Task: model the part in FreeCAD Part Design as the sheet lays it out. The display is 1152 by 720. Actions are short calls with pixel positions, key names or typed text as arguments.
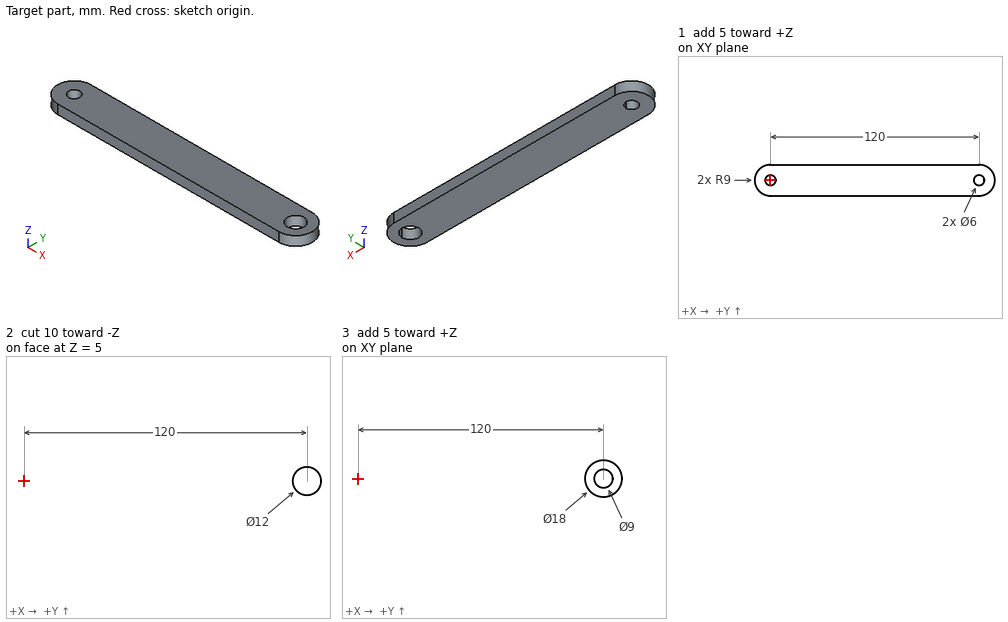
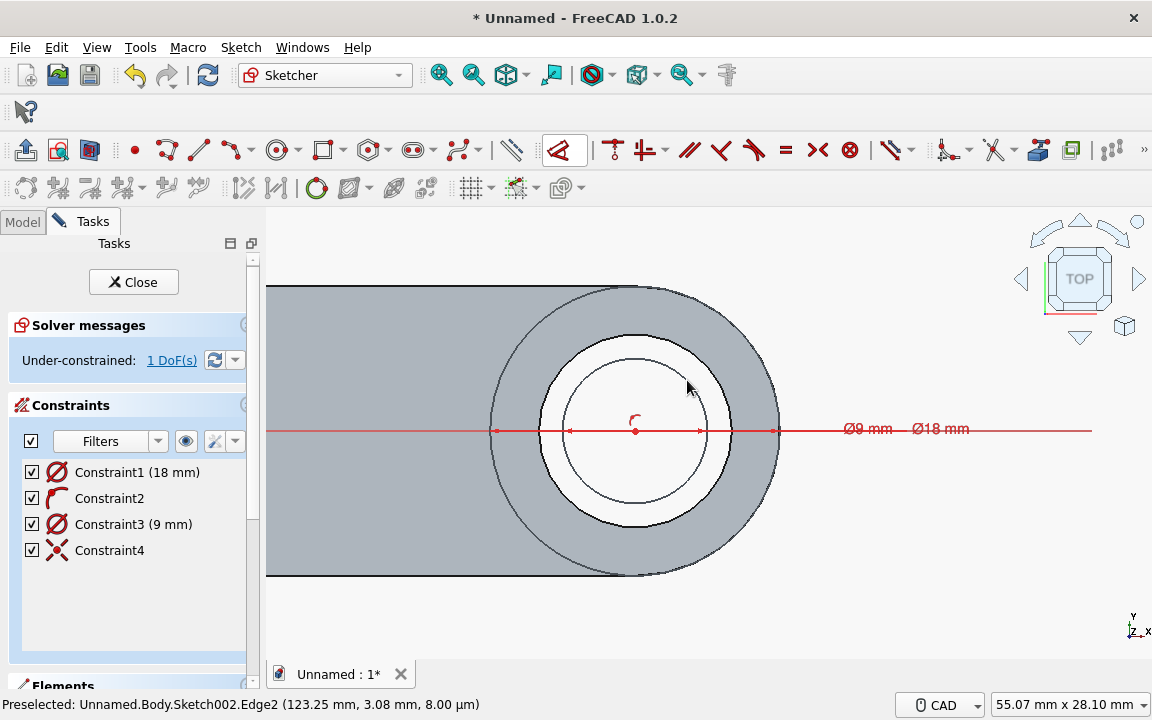
click(635, 431)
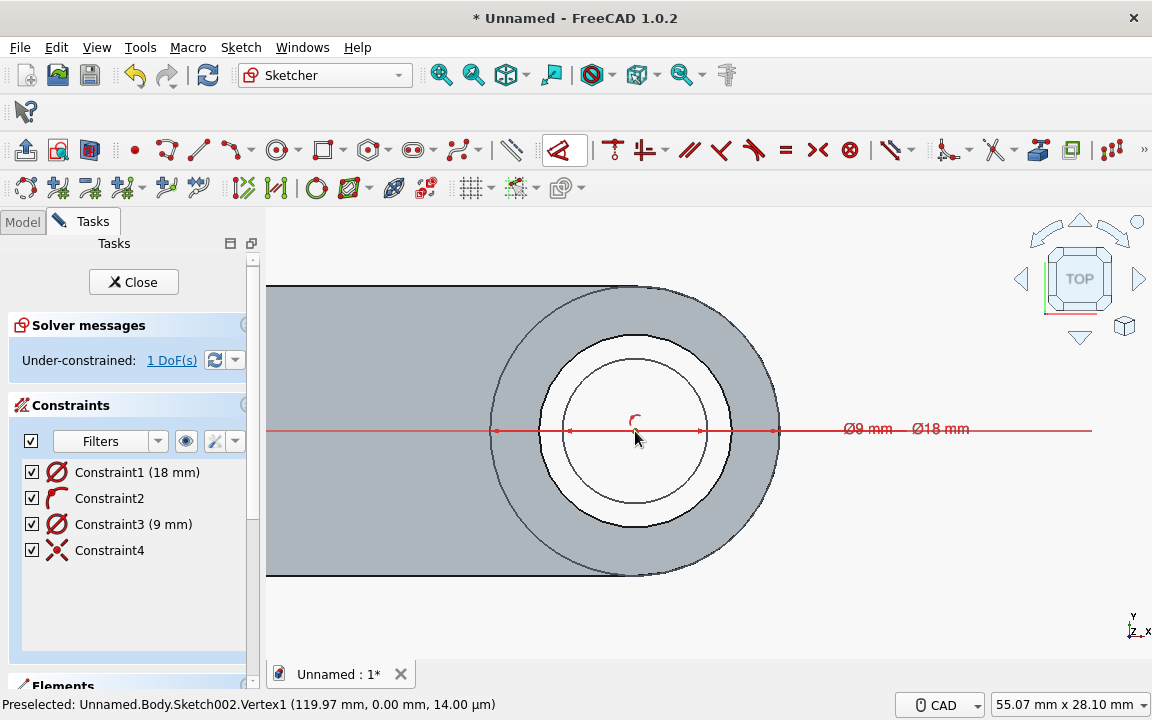
click(582, 150)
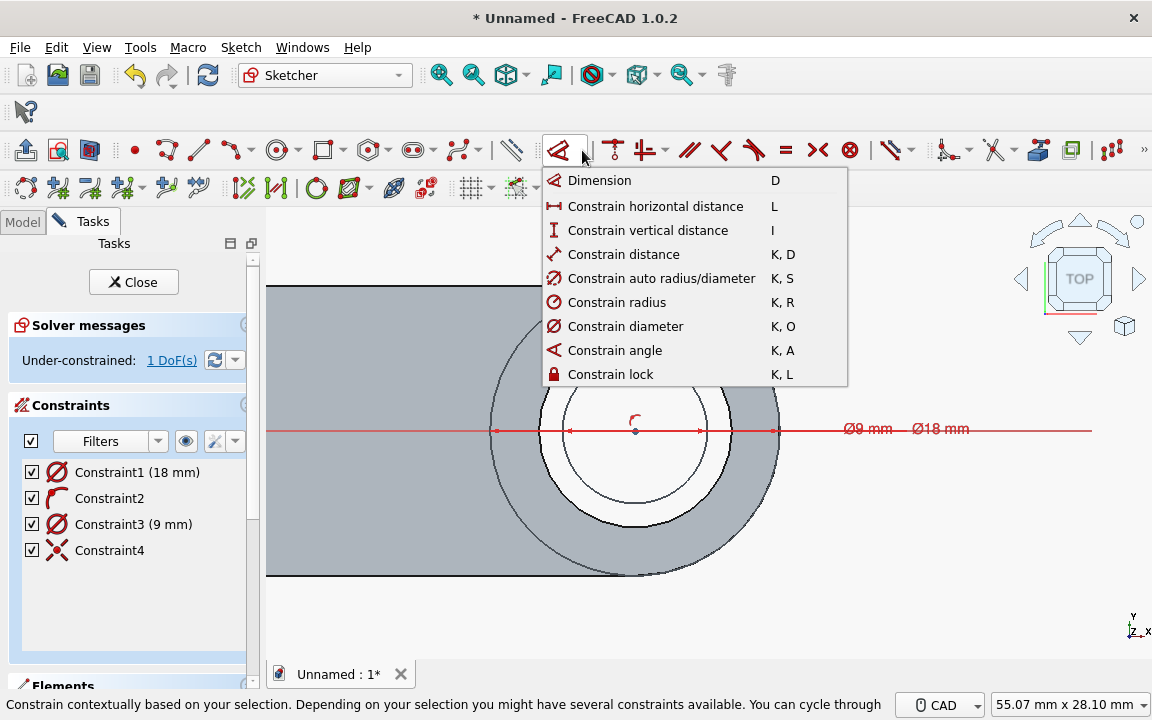
click(695, 206)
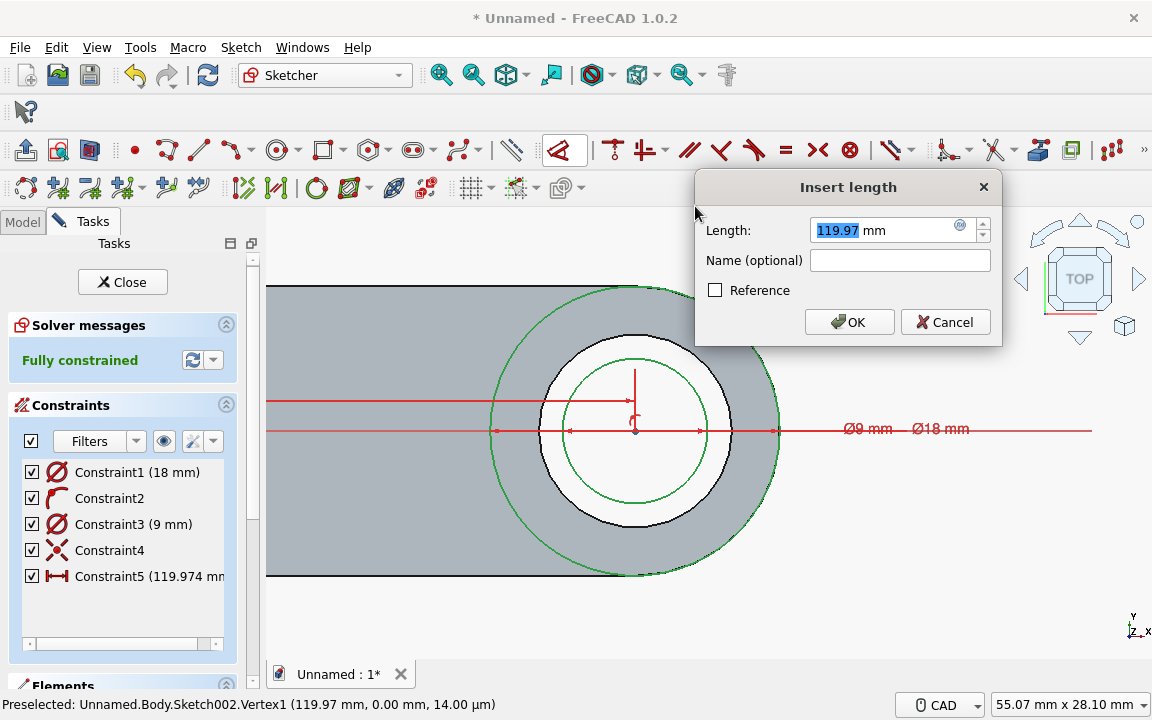
text(120)
key(Return)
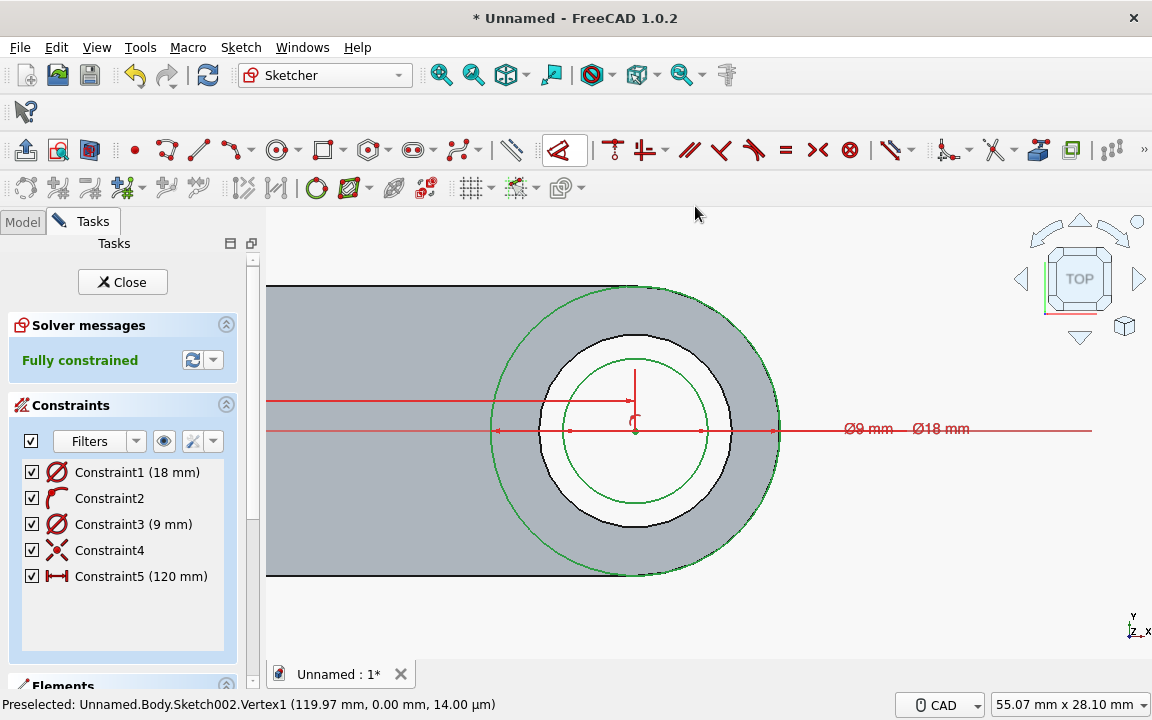
click(123, 282)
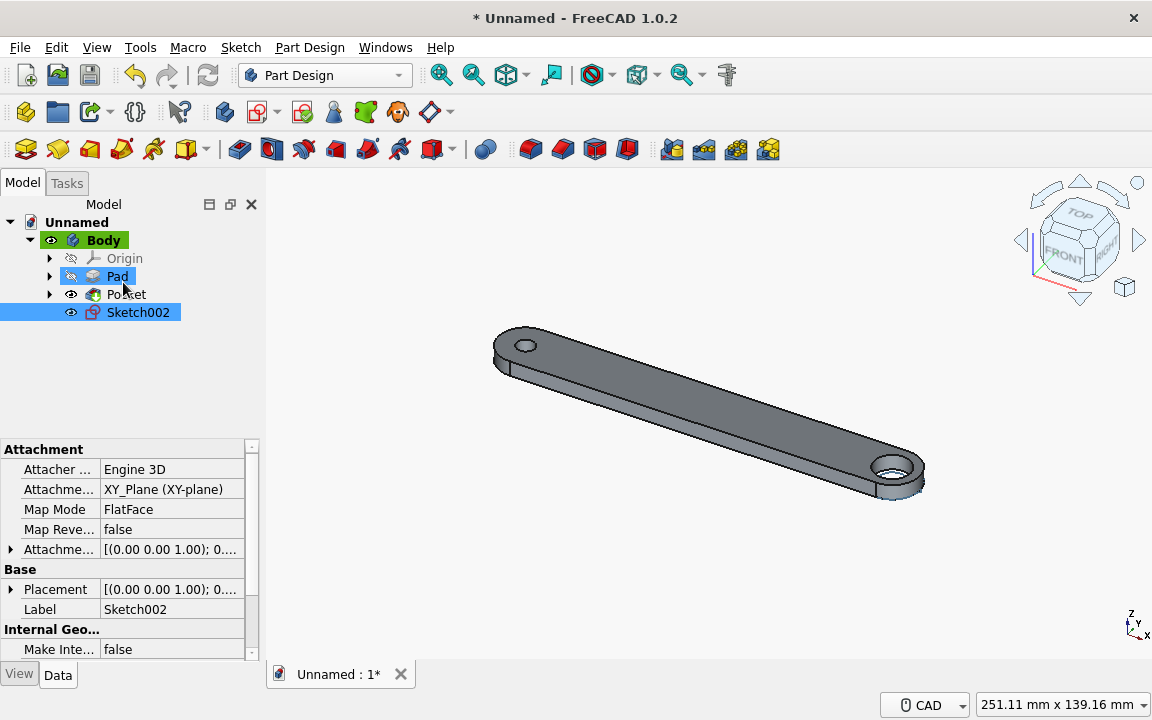
click(26, 150)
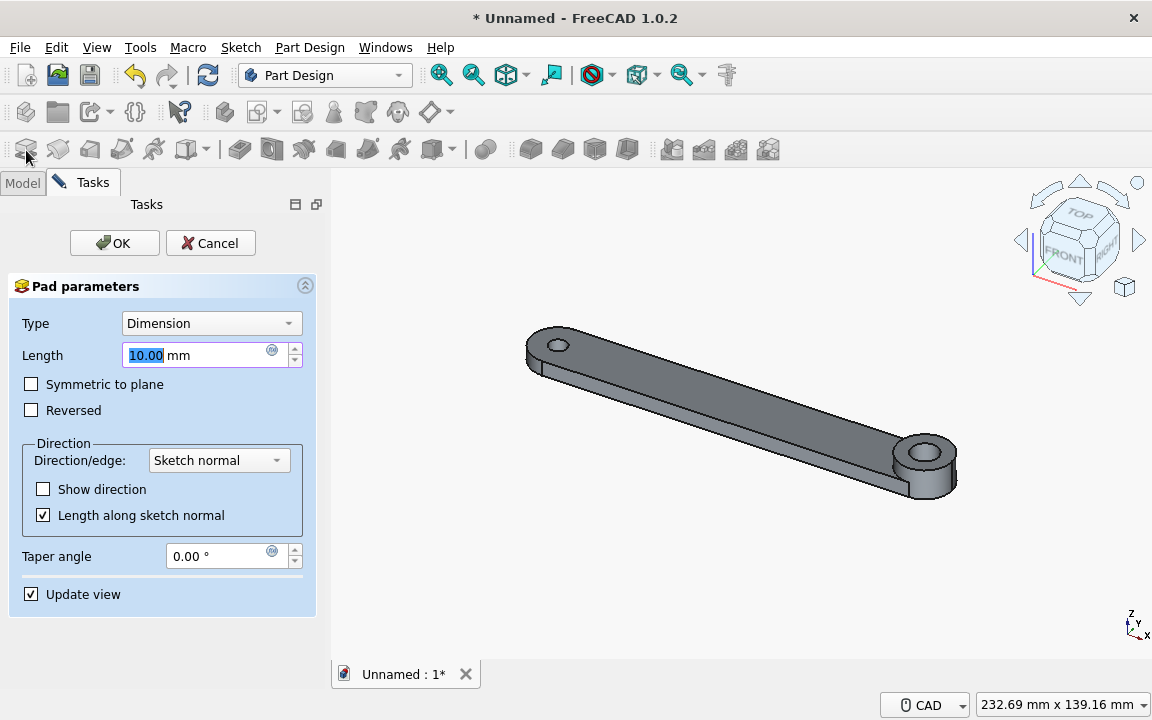
text(5)
key(Tab)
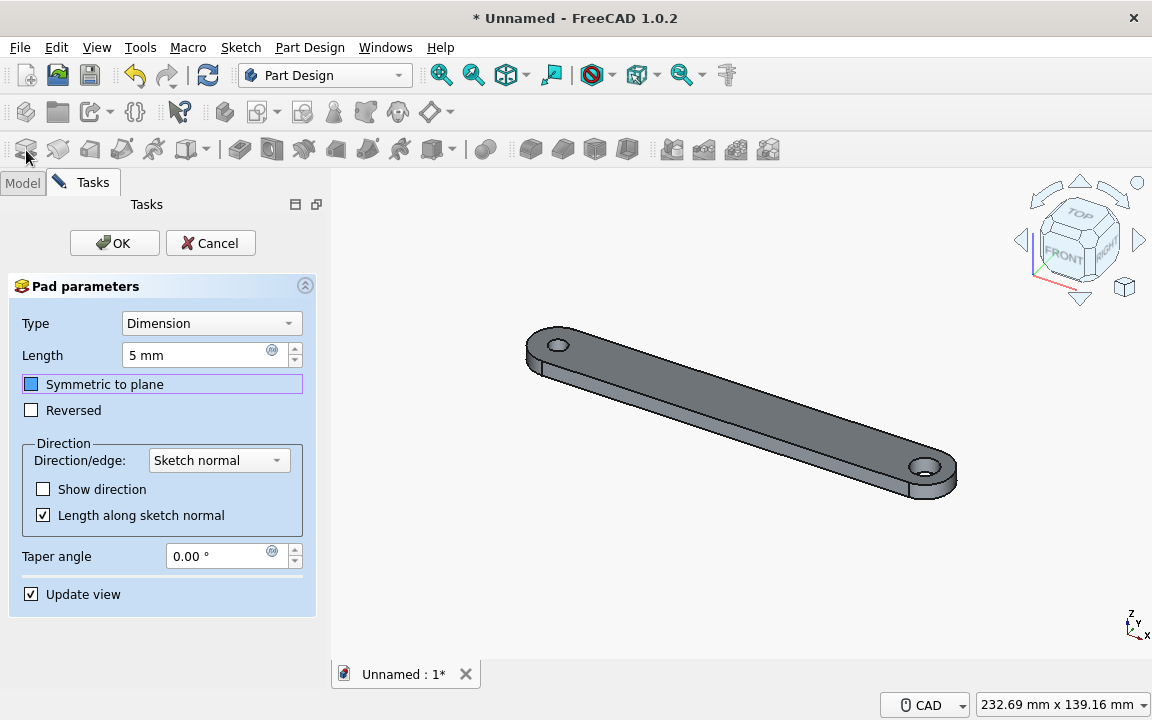
click(115, 243)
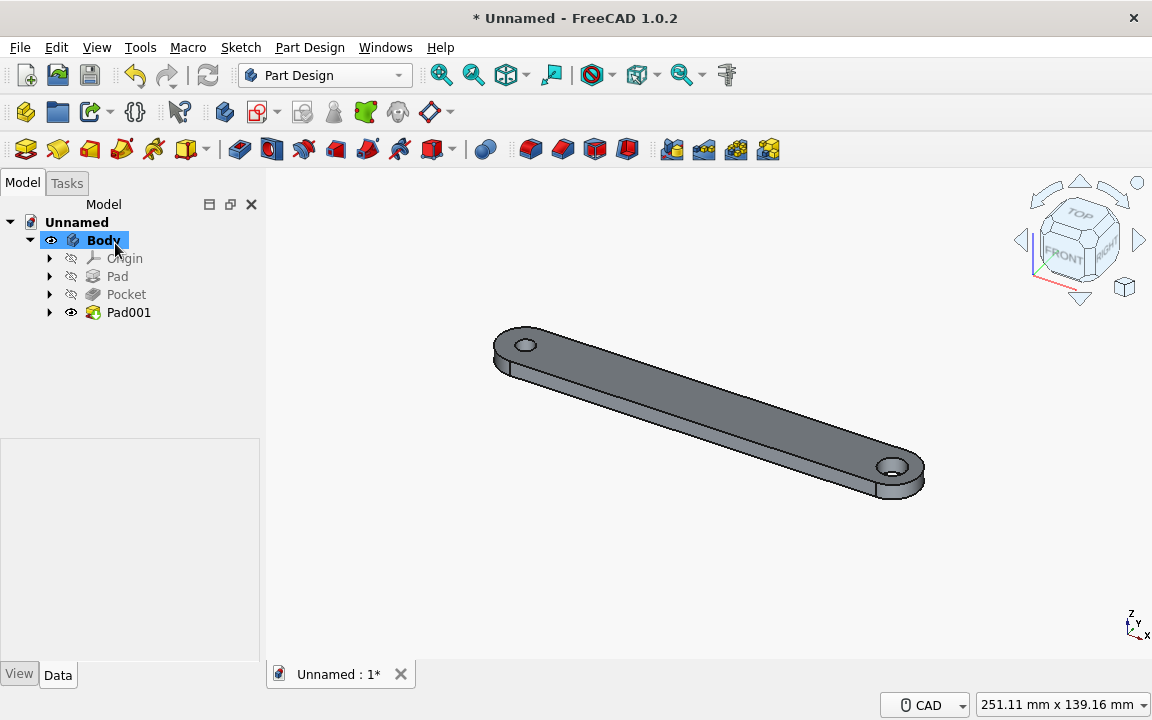
key(0)